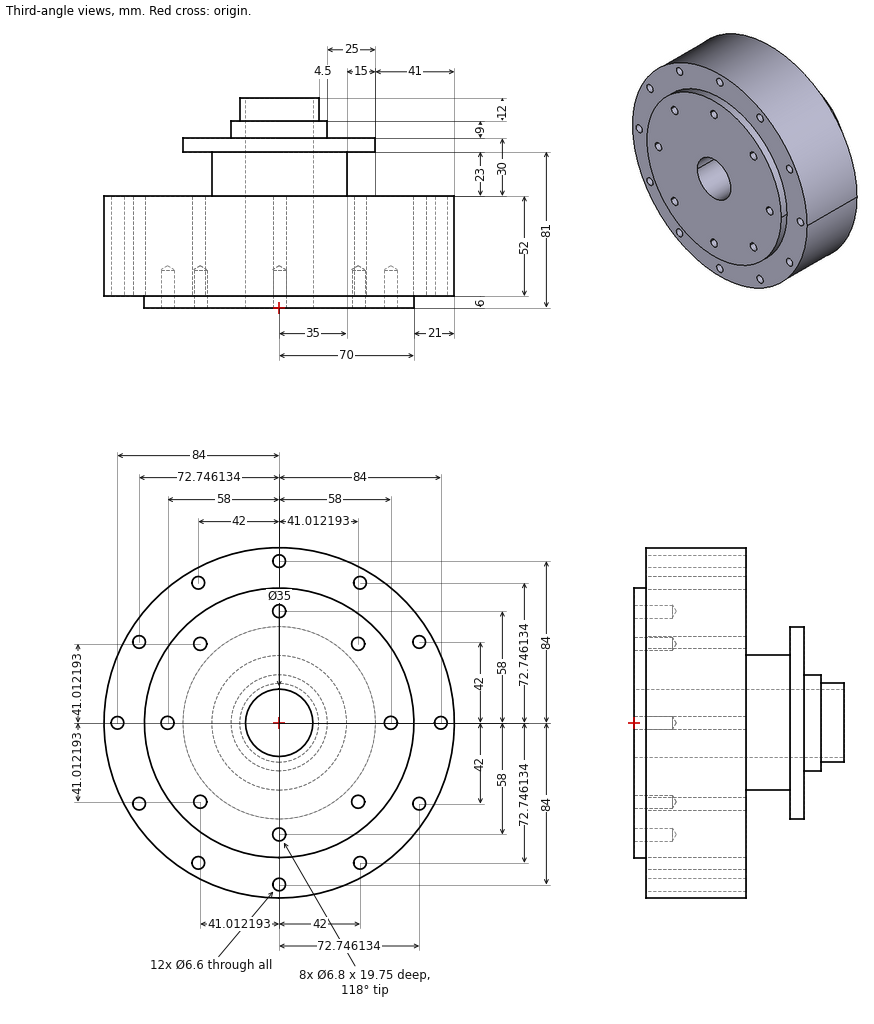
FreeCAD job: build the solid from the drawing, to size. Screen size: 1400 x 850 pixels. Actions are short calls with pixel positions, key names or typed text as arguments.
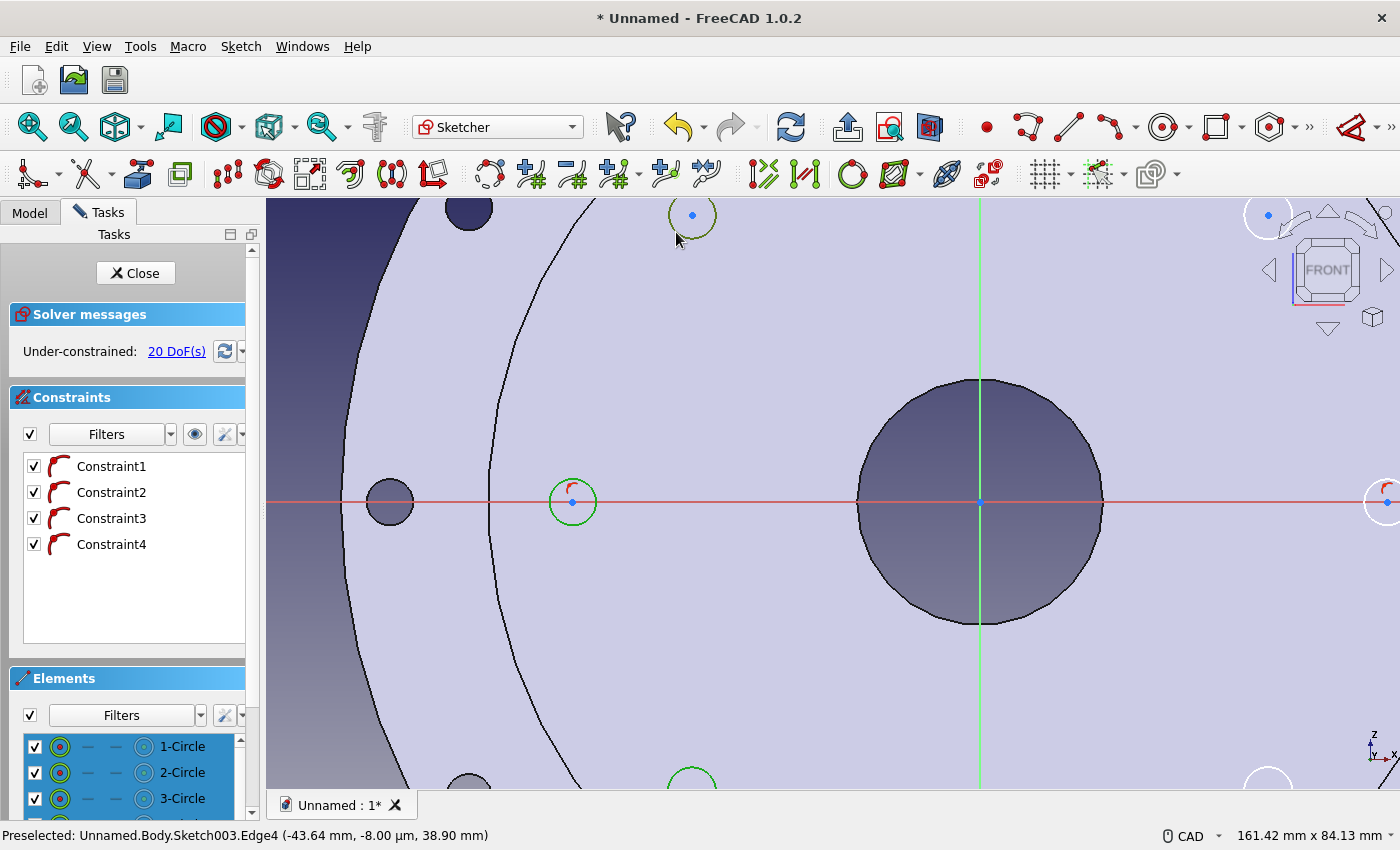
scroll(589, 486, down, 4)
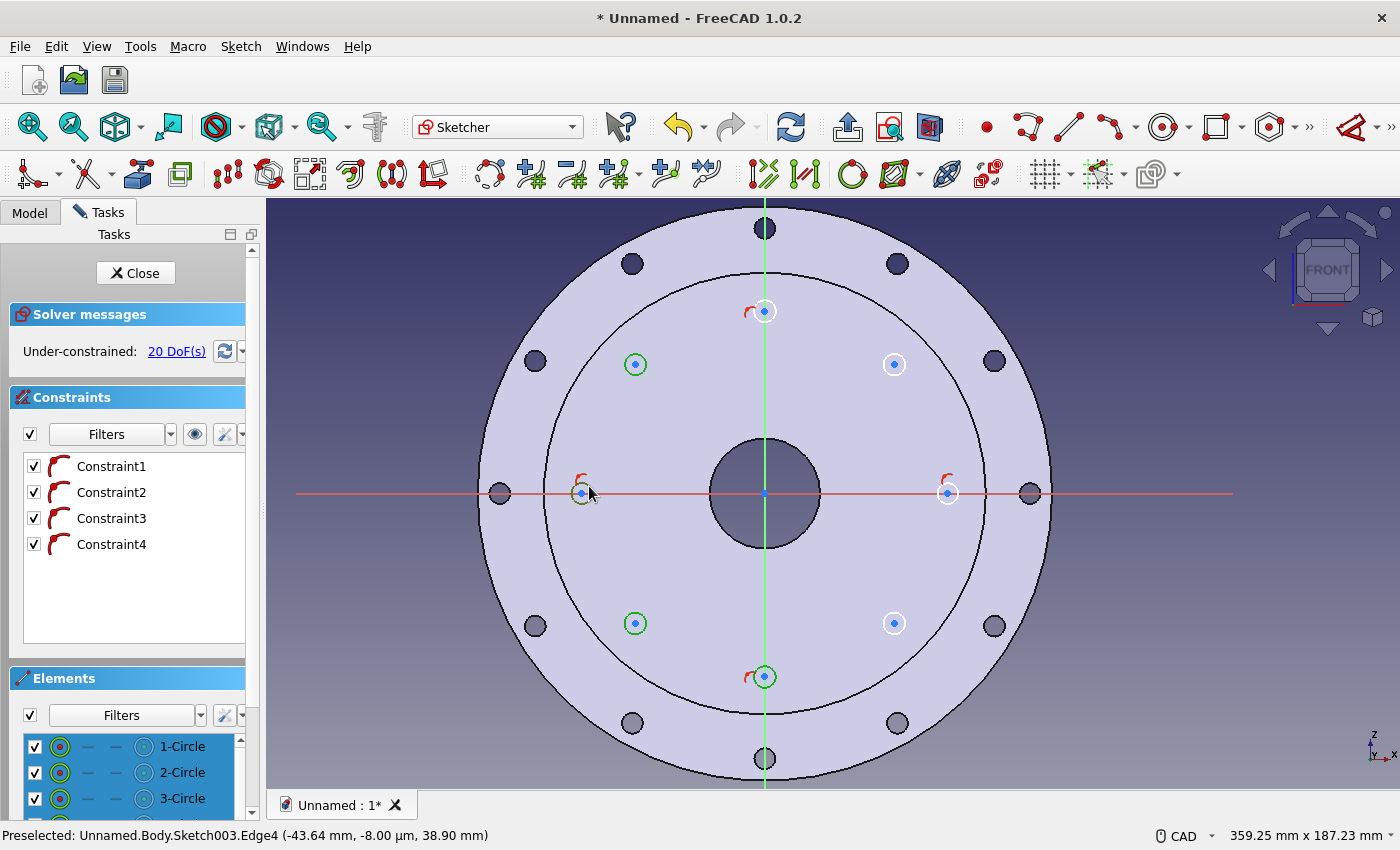
scroll(773, 303, up, 3)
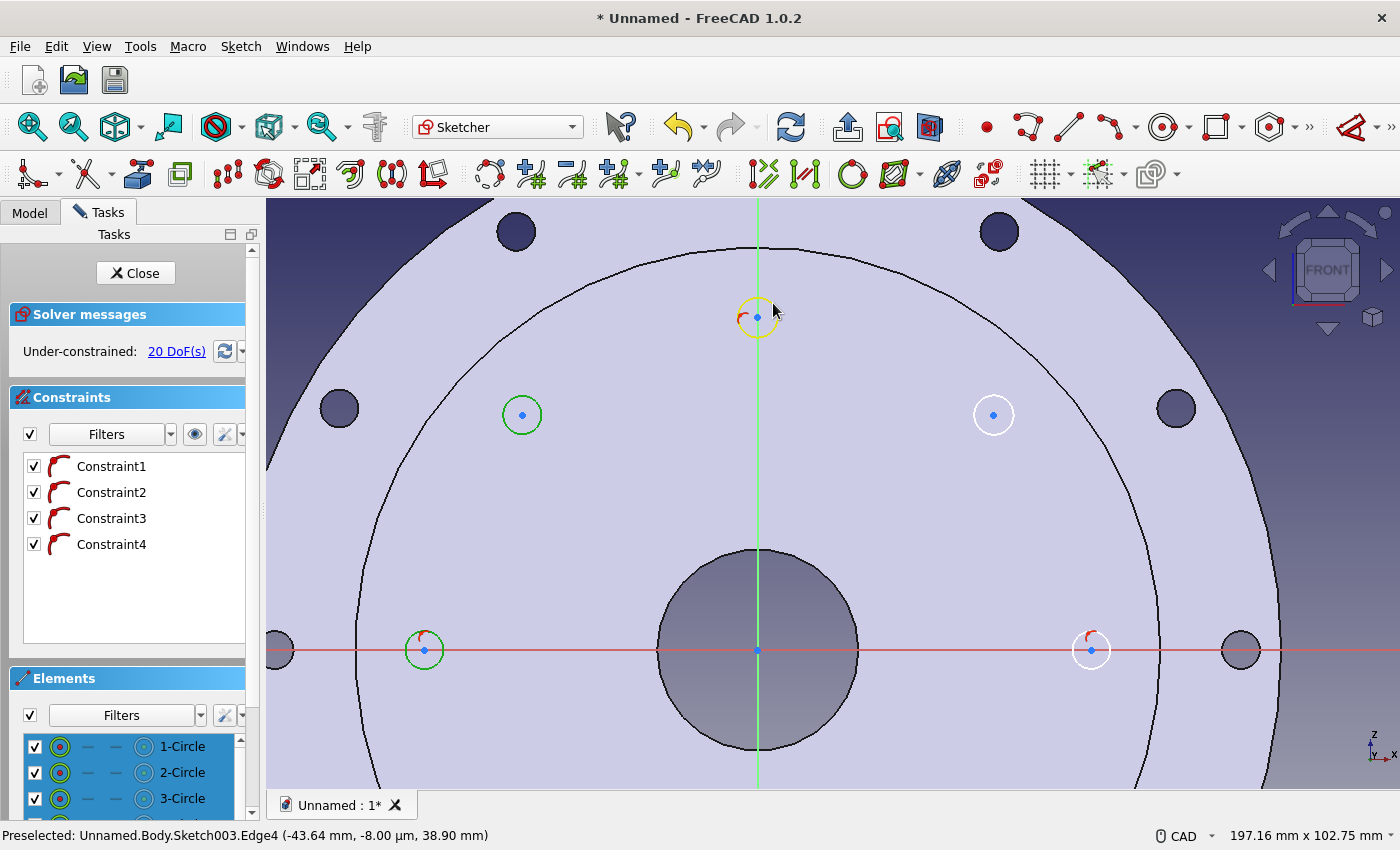
click(772, 304)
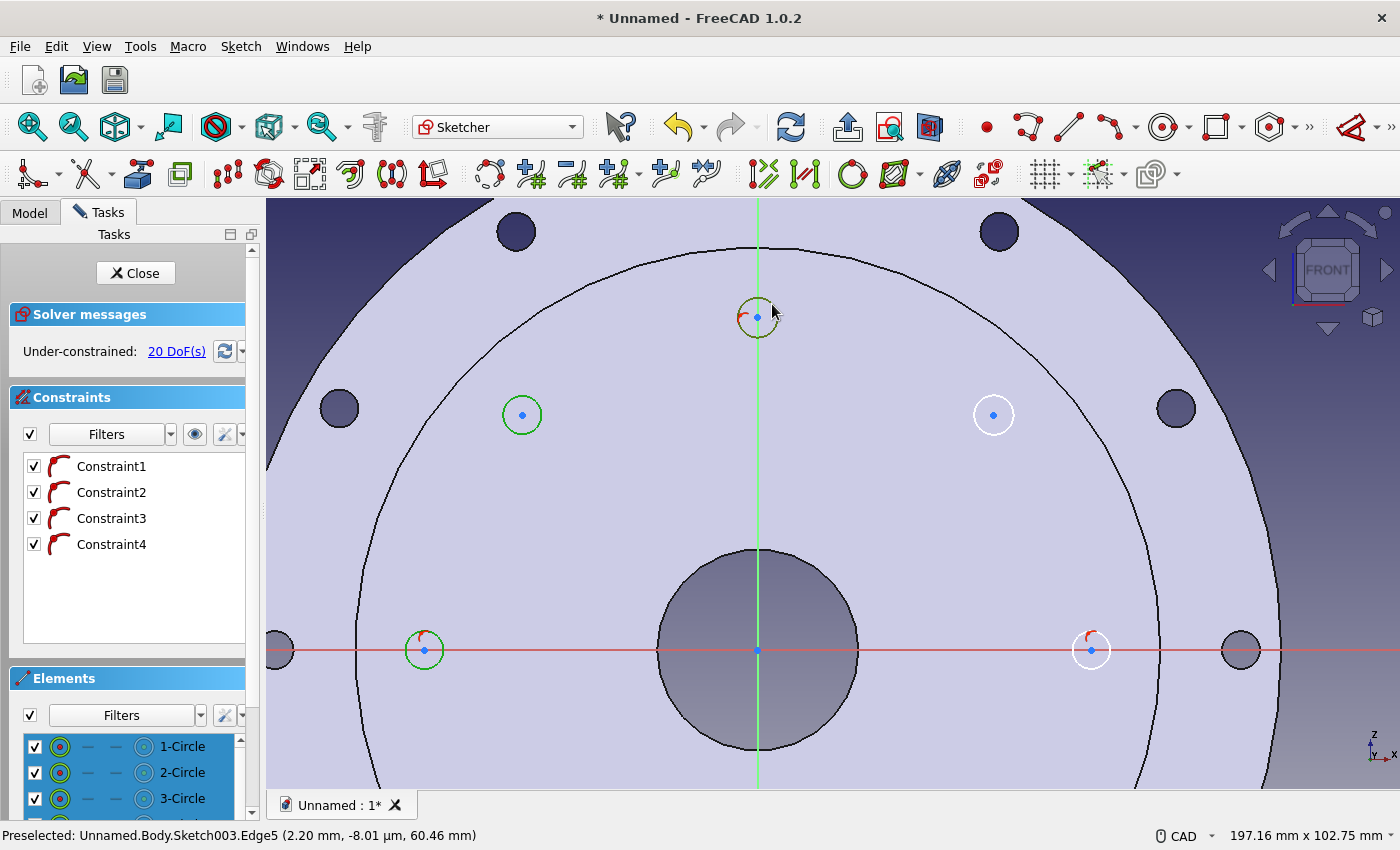
click(1008, 401)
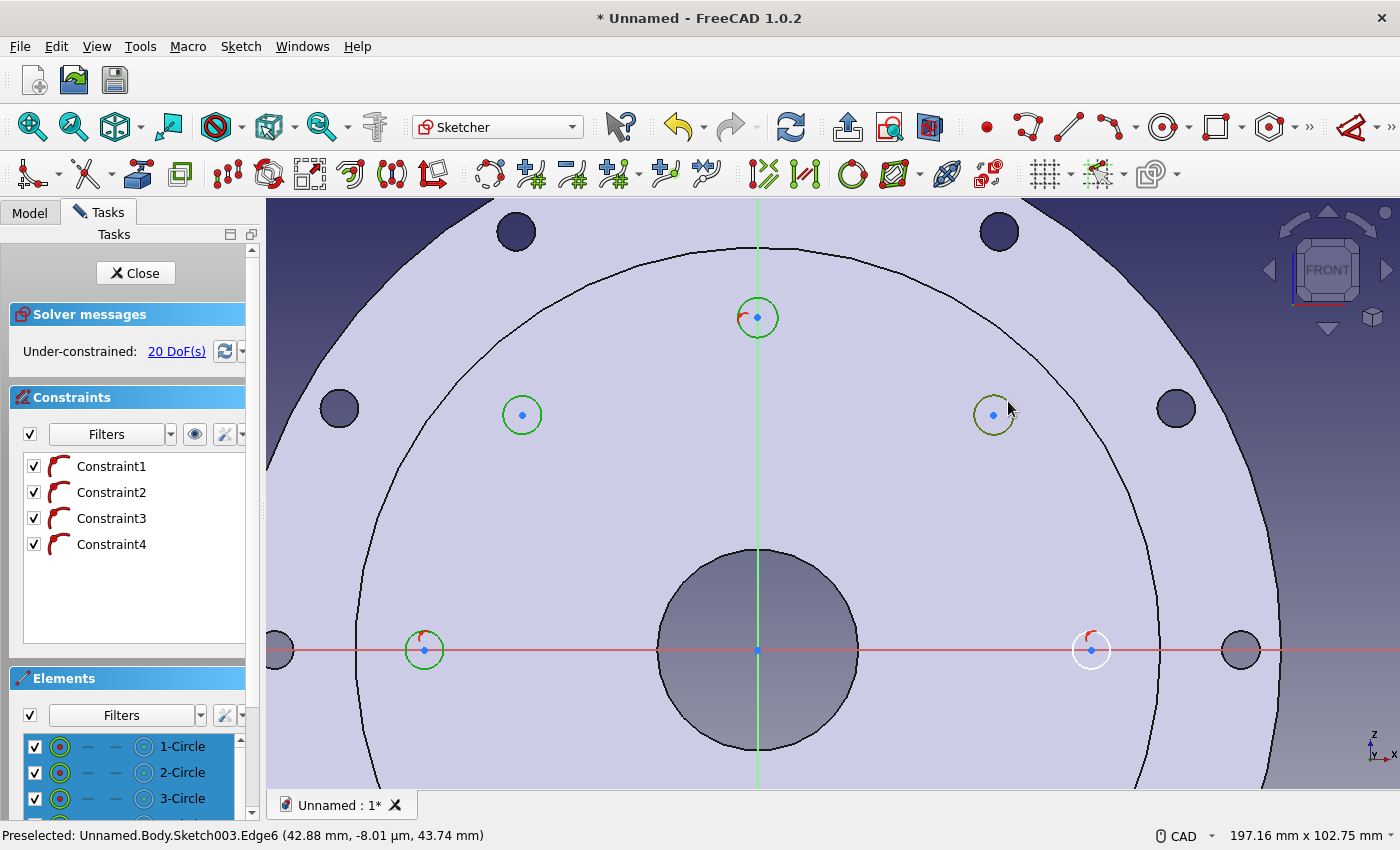
click(1105, 637)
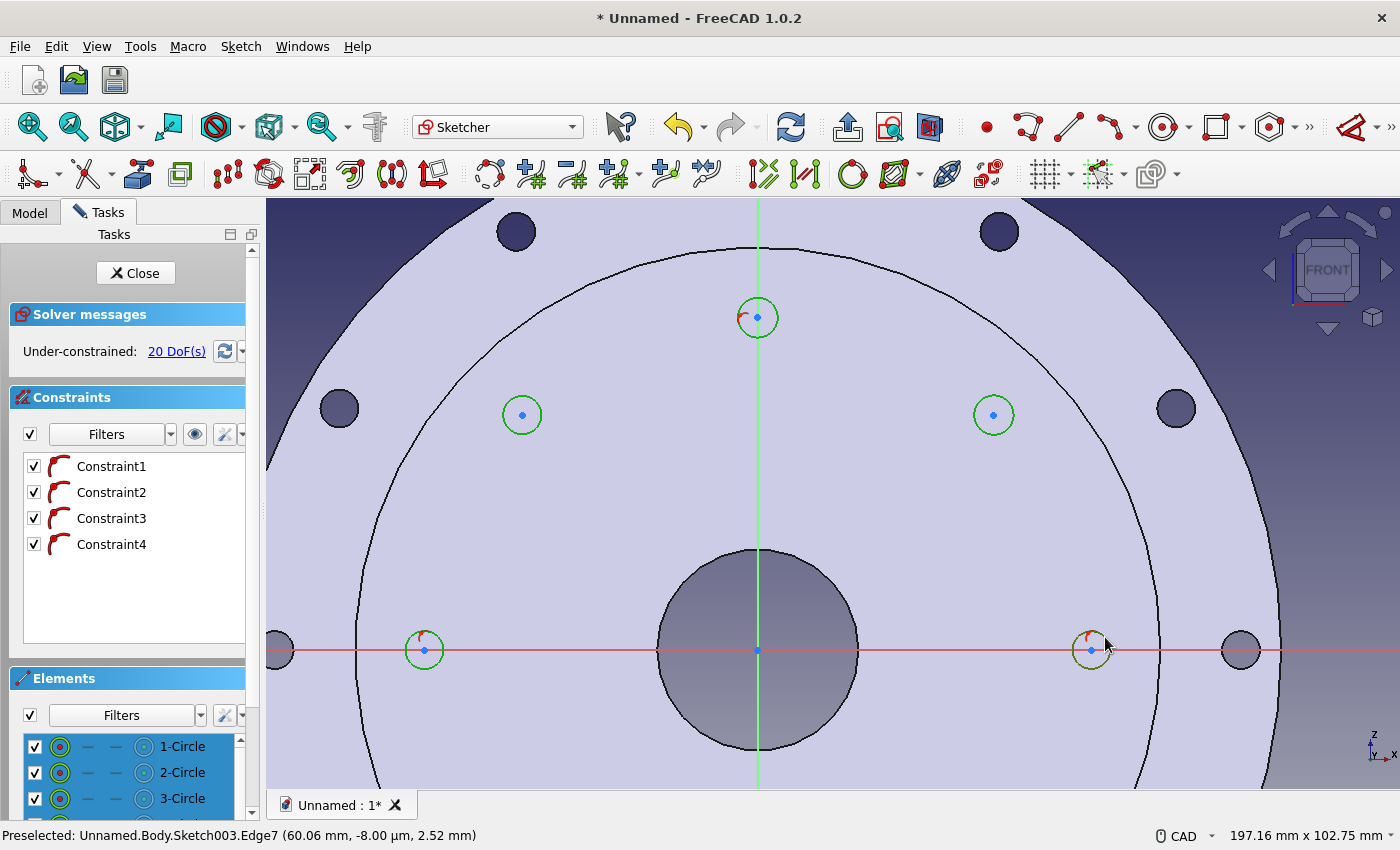
scroll(773, 303, down, 3)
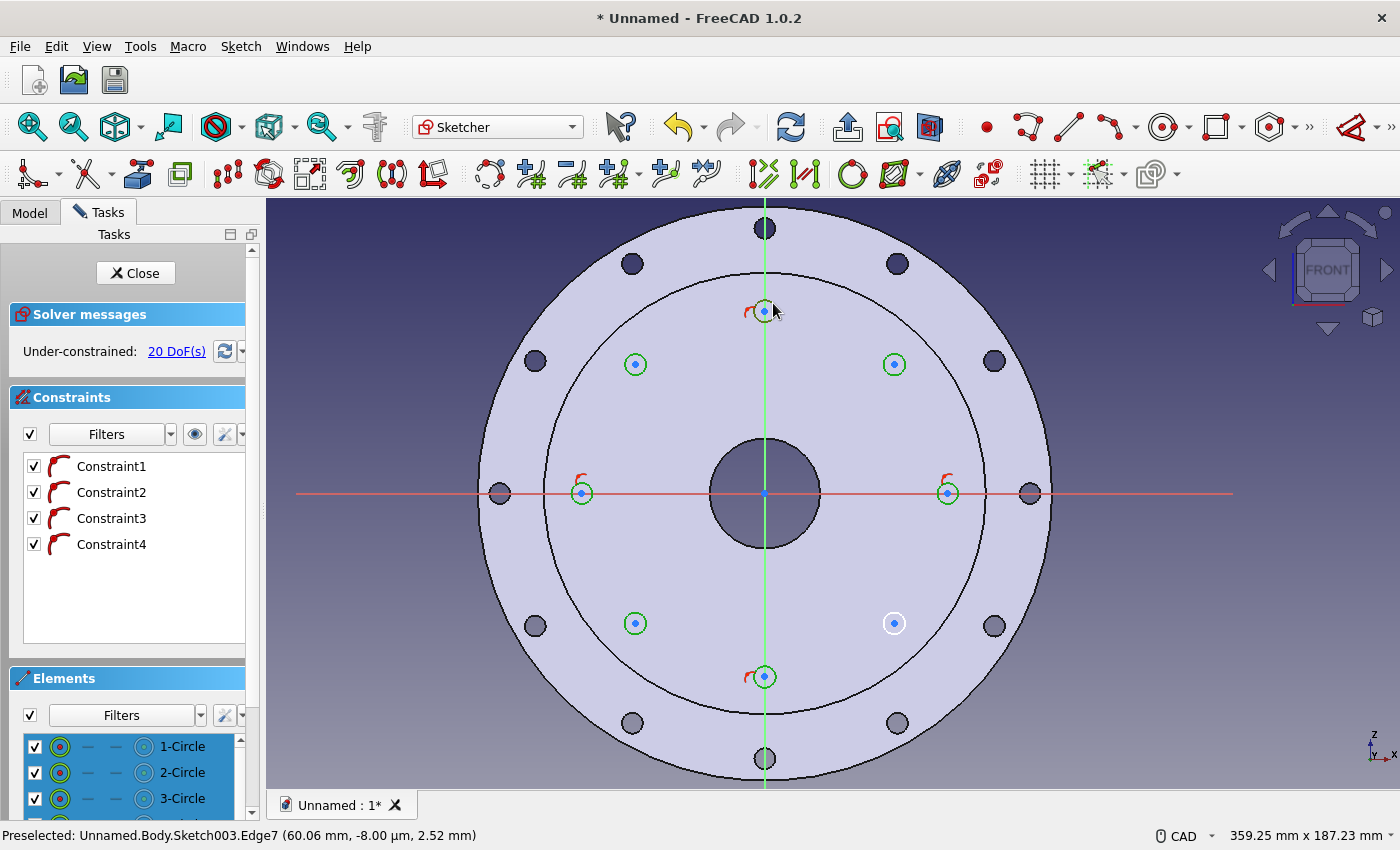
scroll(902, 616, up, 2)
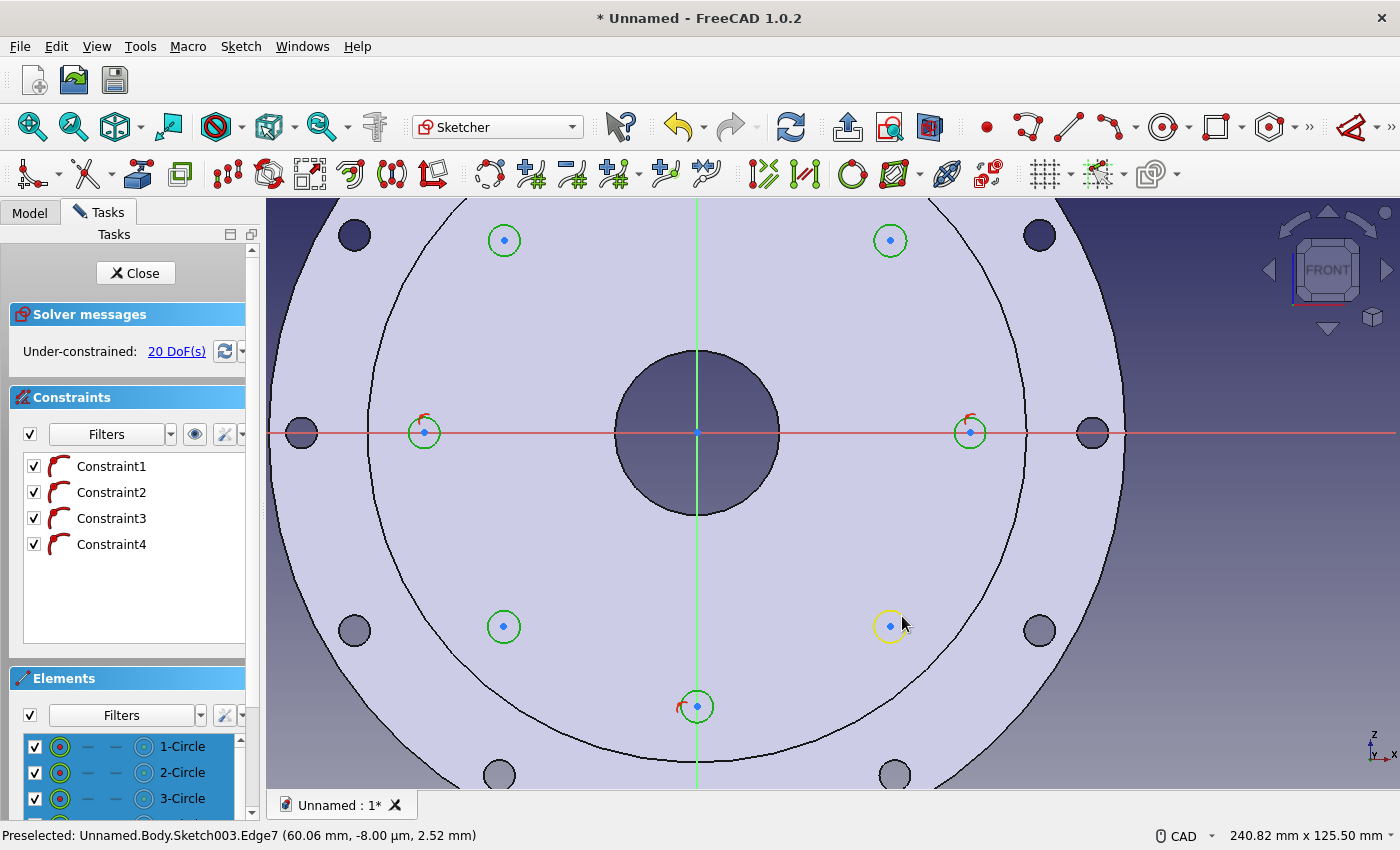
click(902, 615)